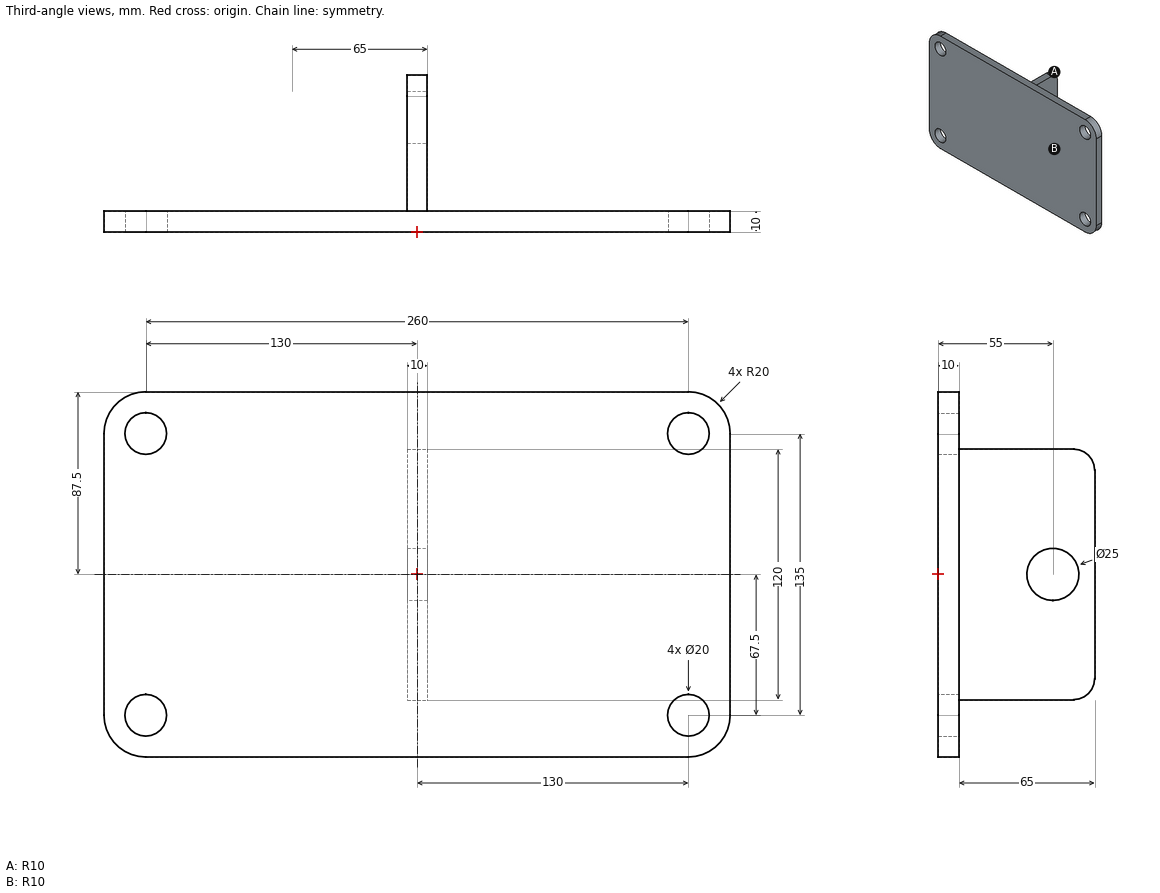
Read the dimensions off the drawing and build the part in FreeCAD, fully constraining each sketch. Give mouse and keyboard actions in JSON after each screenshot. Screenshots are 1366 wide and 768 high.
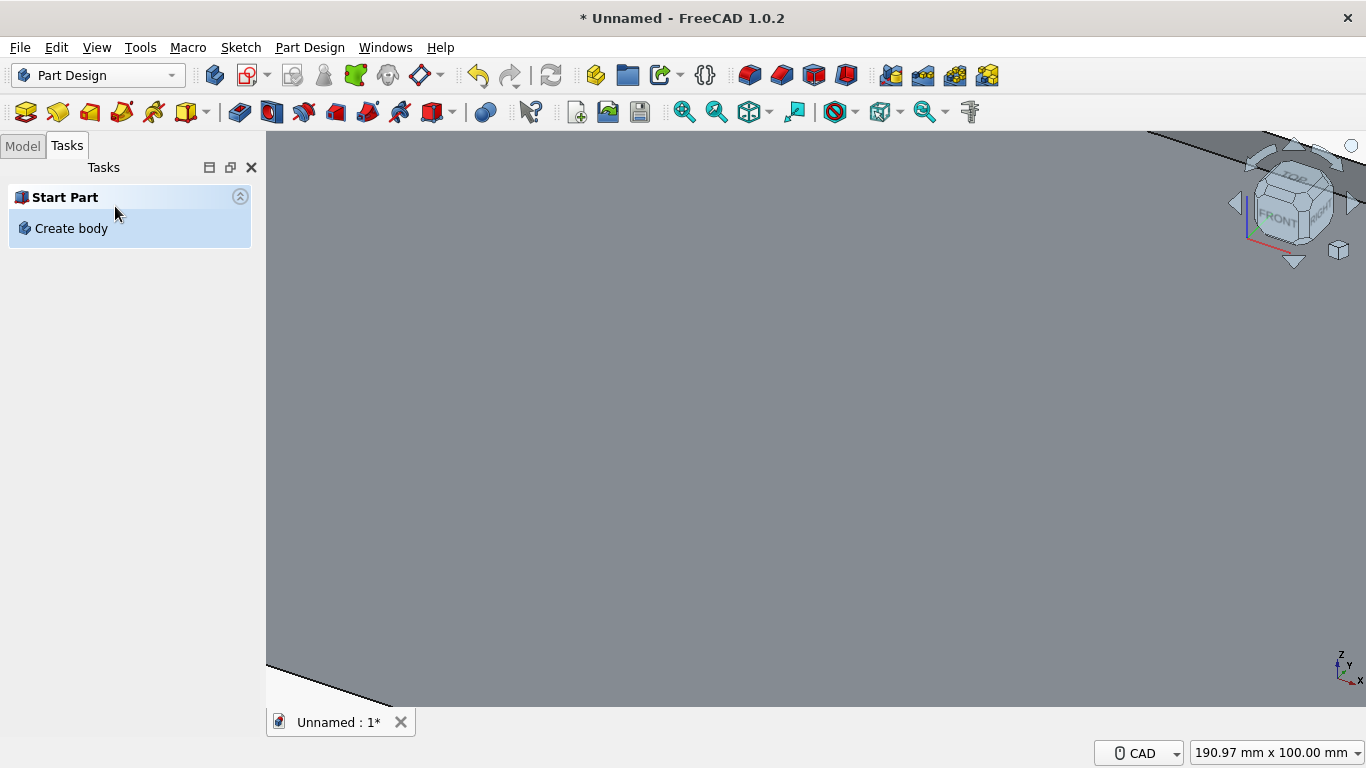
{"action": "left_click", "coordinate": [686, 112]}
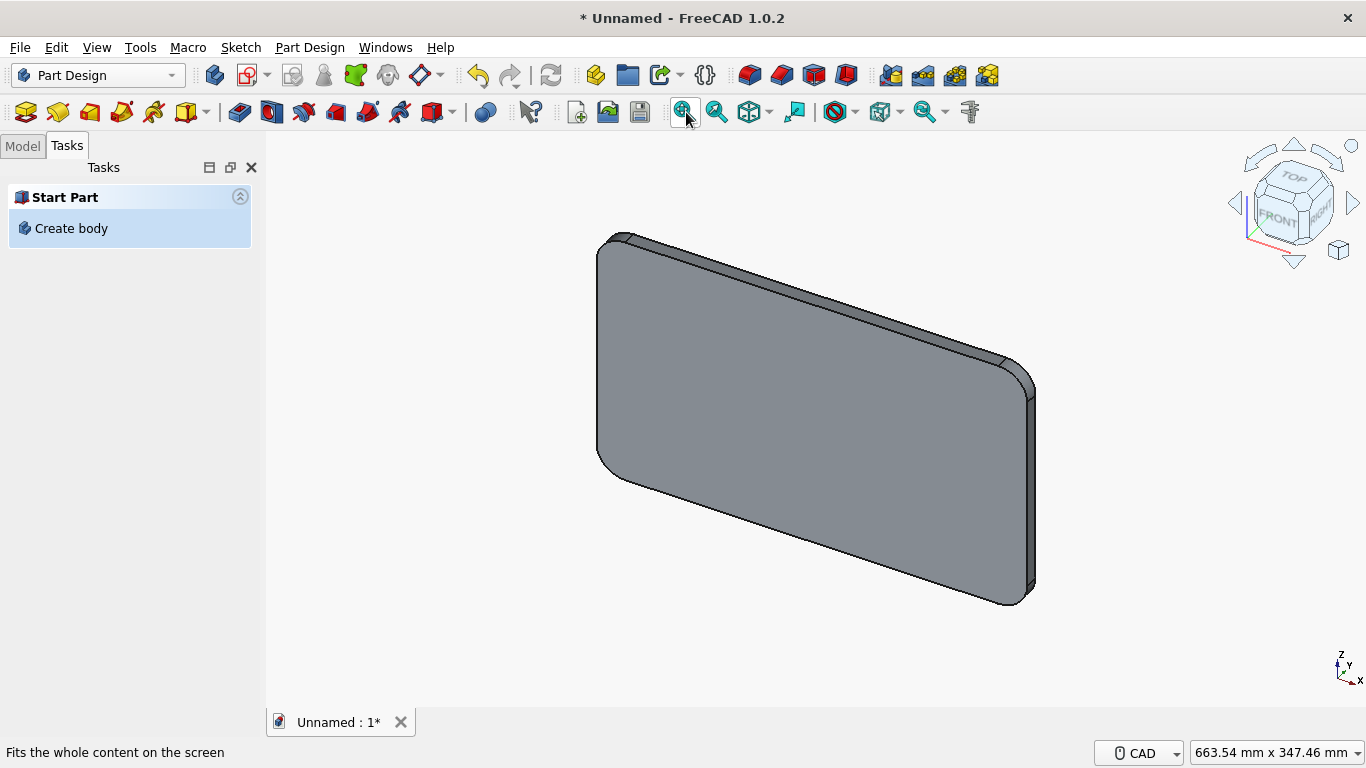
{"action": "key", "text": "4"}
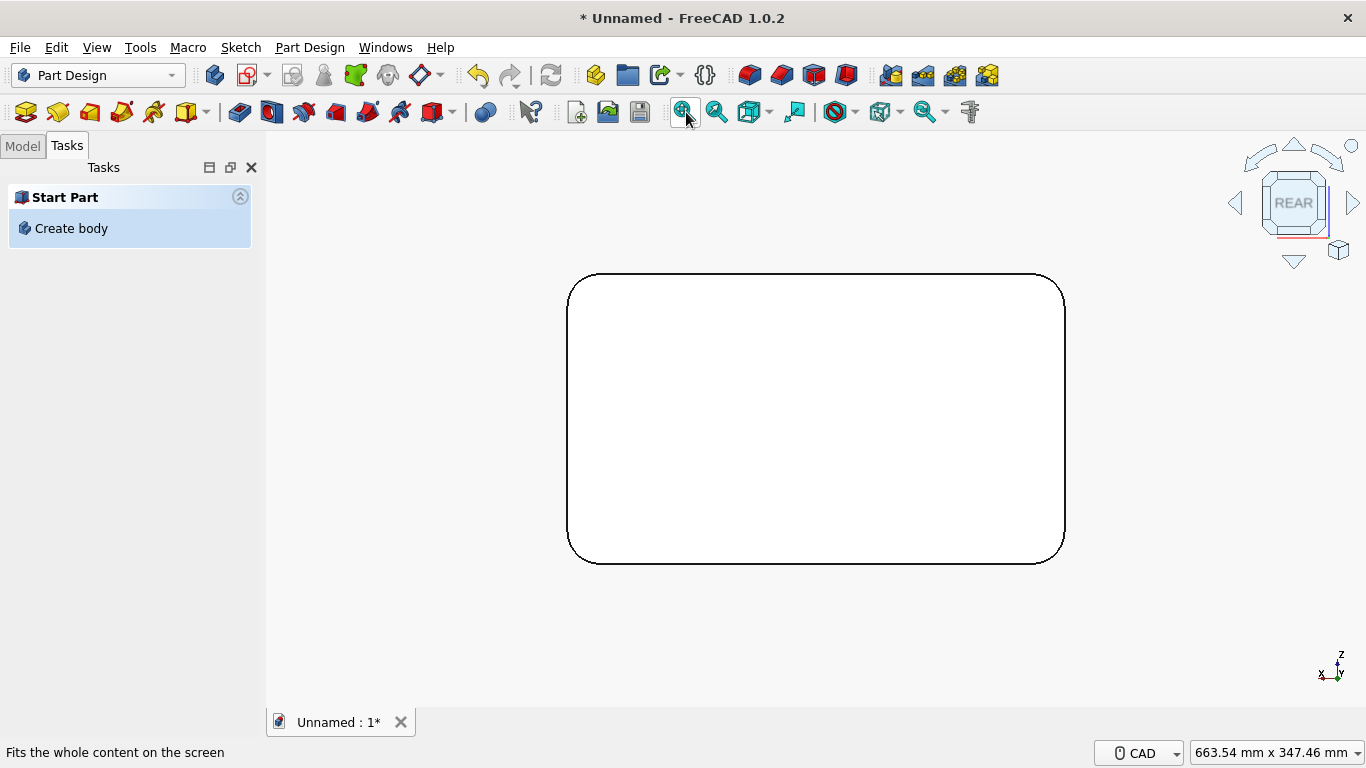
{"action": "left_click", "coordinate": [745, 418]}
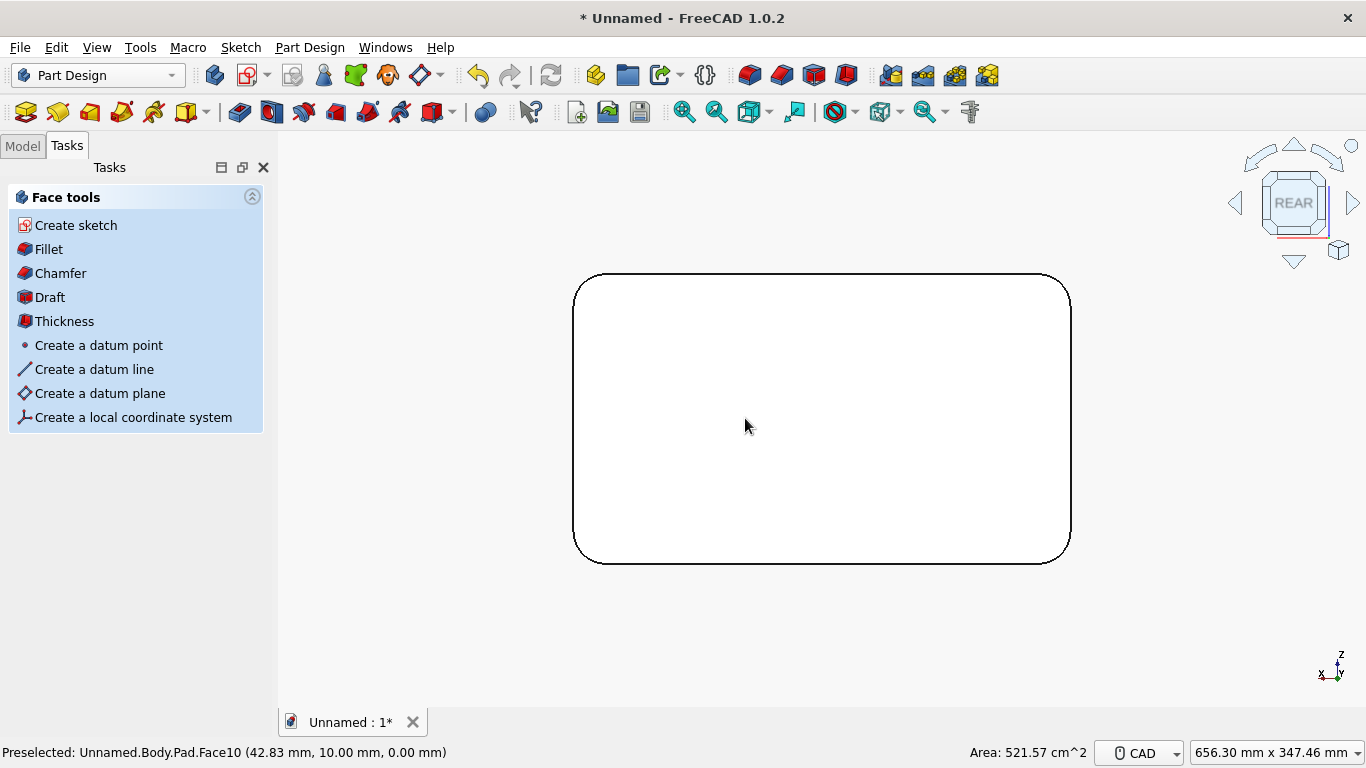
{"action": "left_click", "coordinate": [248, 76]}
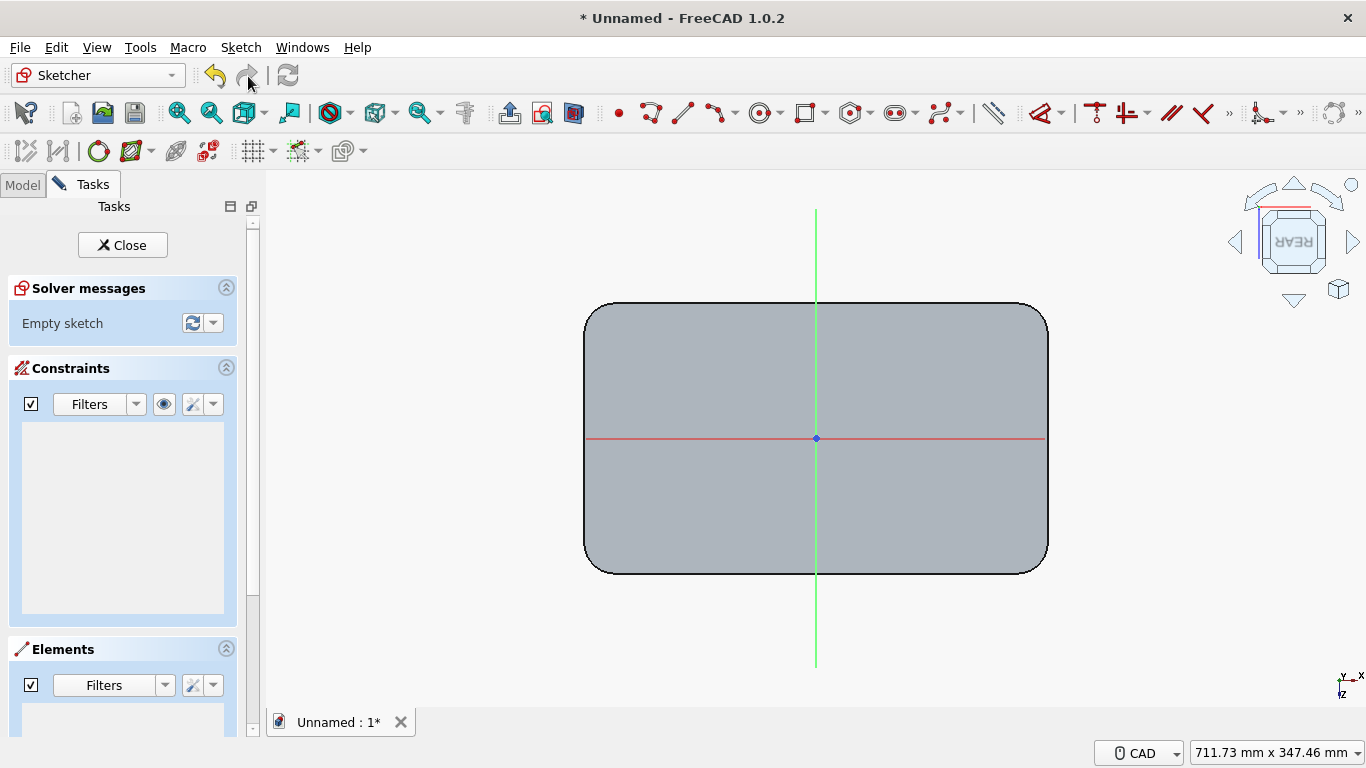
{"action": "scroll", "coordinate": [955, 439], "scroll_direction": "up", "scroll_amount": 2}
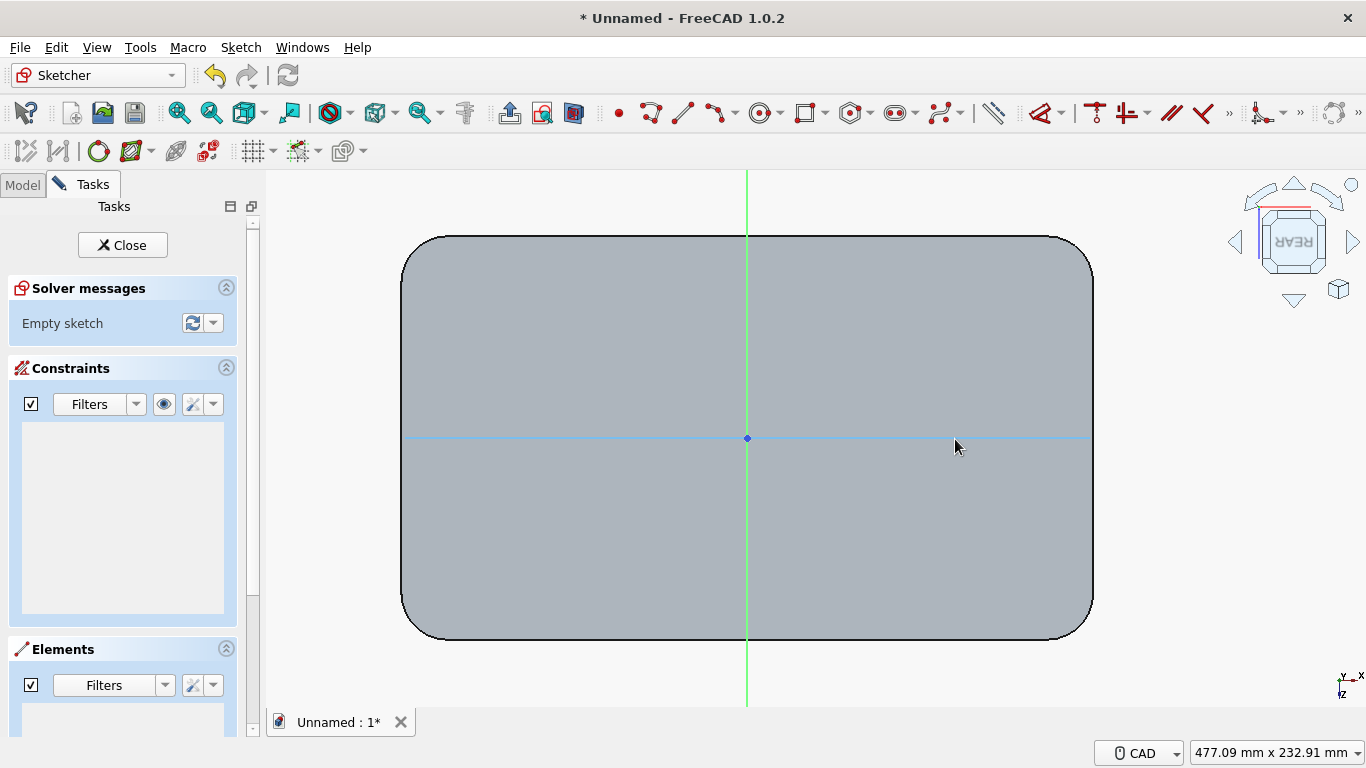
{"action": "left_click", "coordinate": [760, 114]}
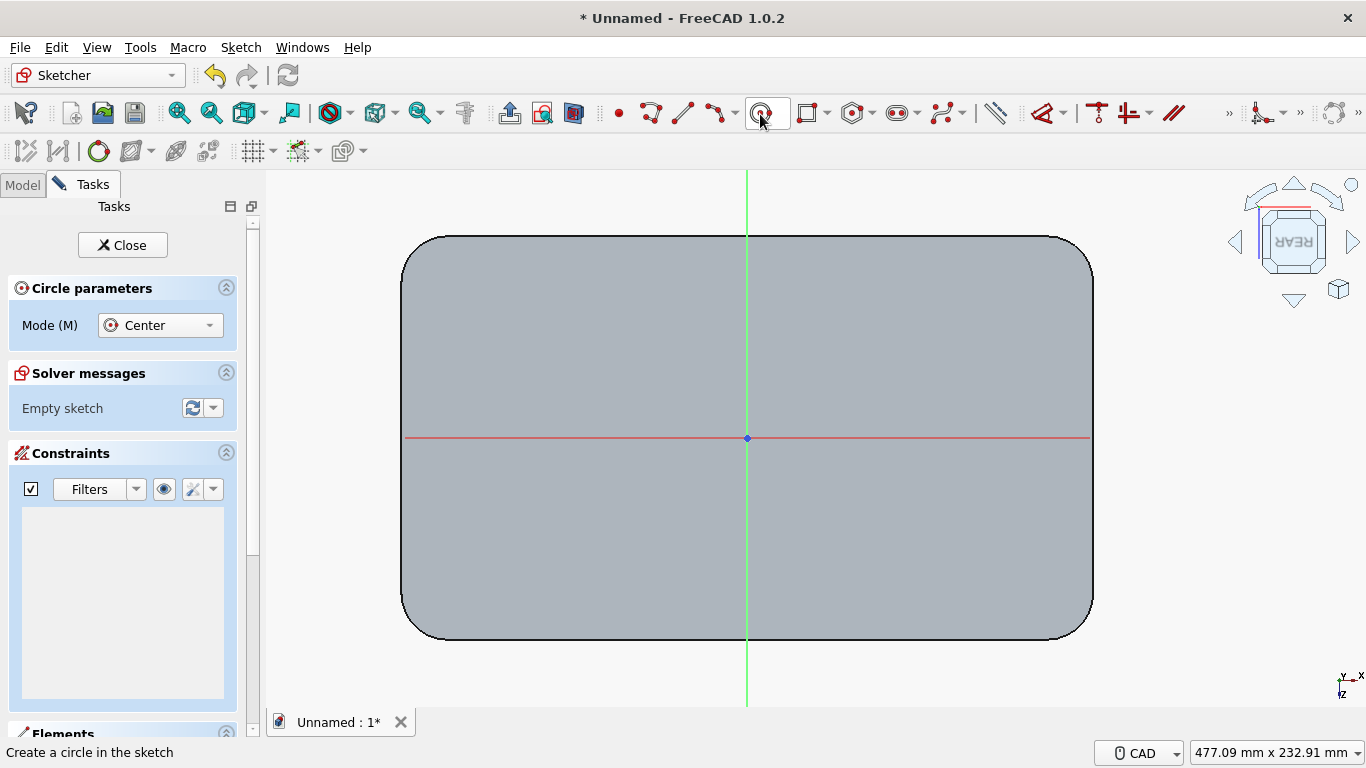
{"action": "left_click", "coordinate": [1047, 282]}
{"action": "left_click", "coordinate": [1063, 266]}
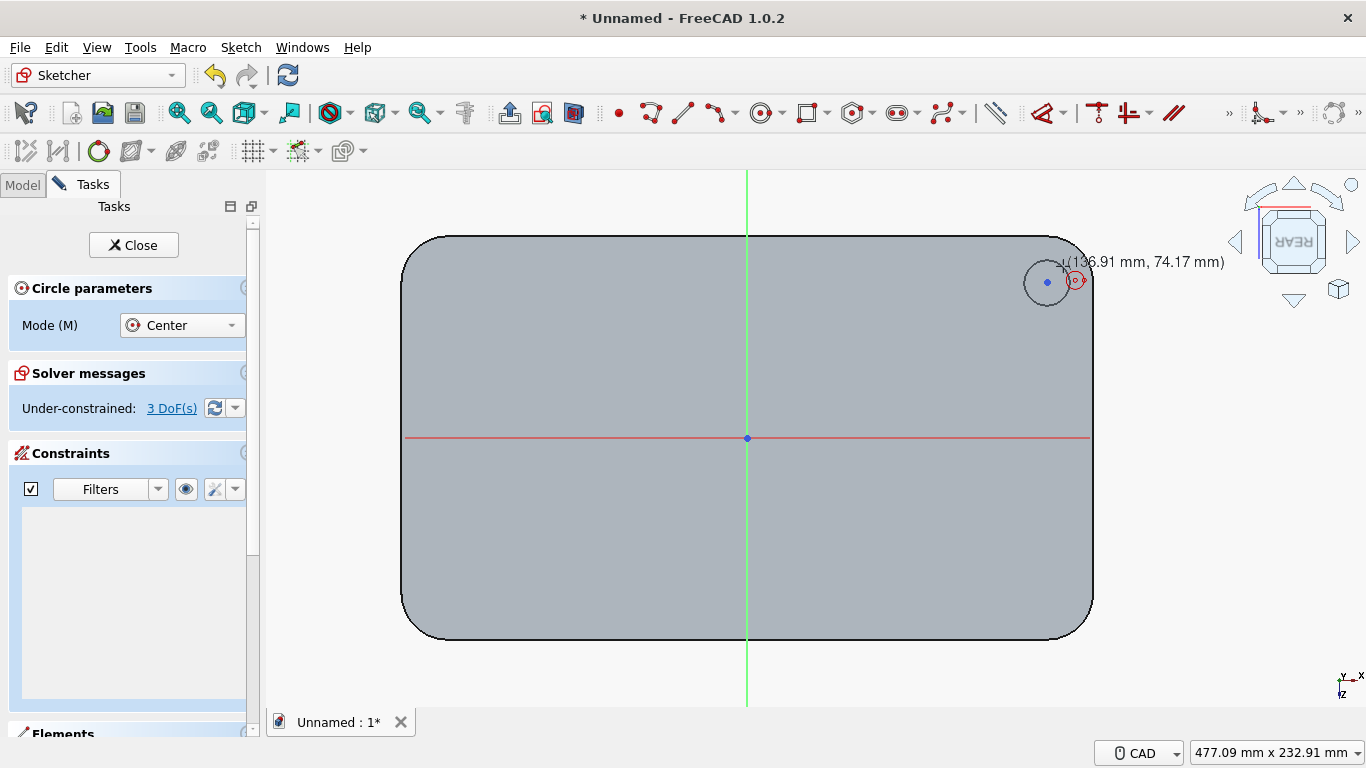
{"action": "left_click", "coordinate": [1047, 594]}
{"action": "left_click", "coordinate": [1063, 577]}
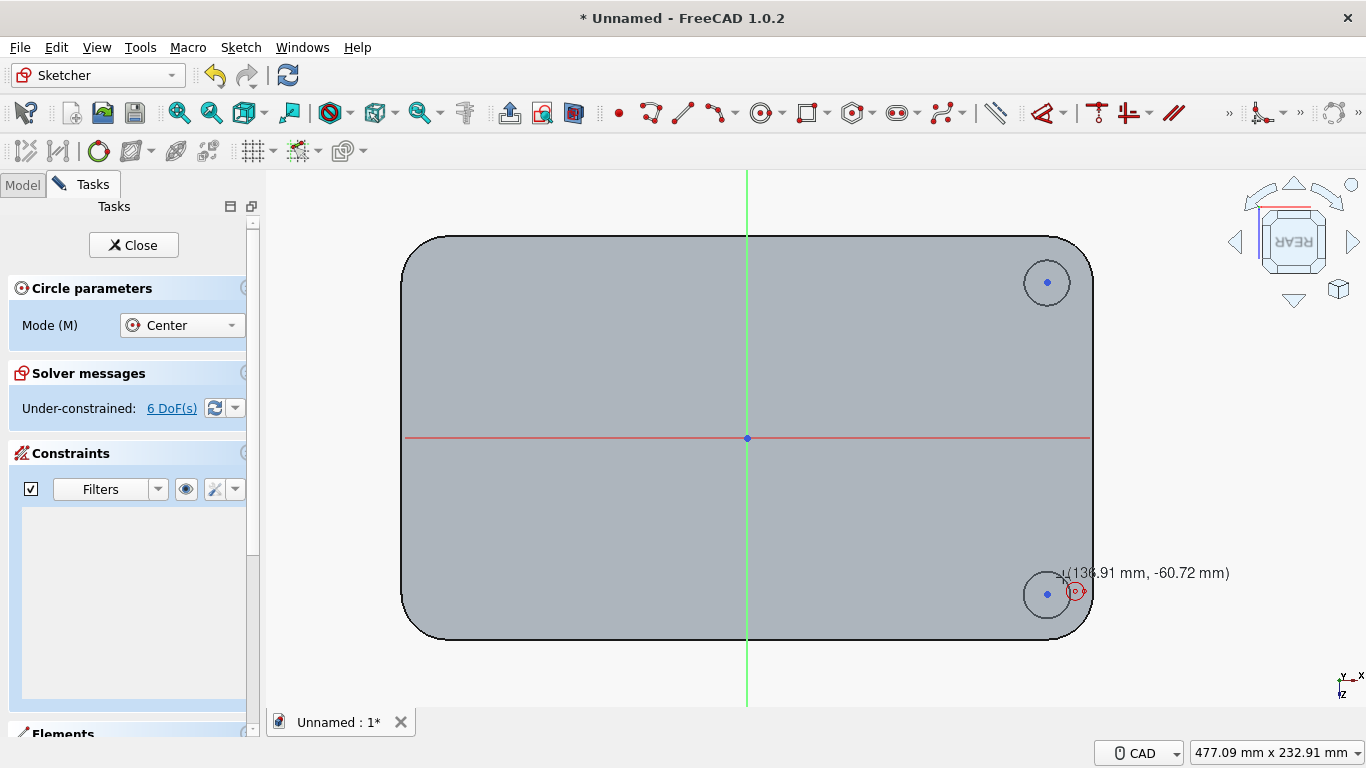
{"action": "left_click", "coordinate": [448, 282]}
{"action": "left_click", "coordinate": [464, 266]}